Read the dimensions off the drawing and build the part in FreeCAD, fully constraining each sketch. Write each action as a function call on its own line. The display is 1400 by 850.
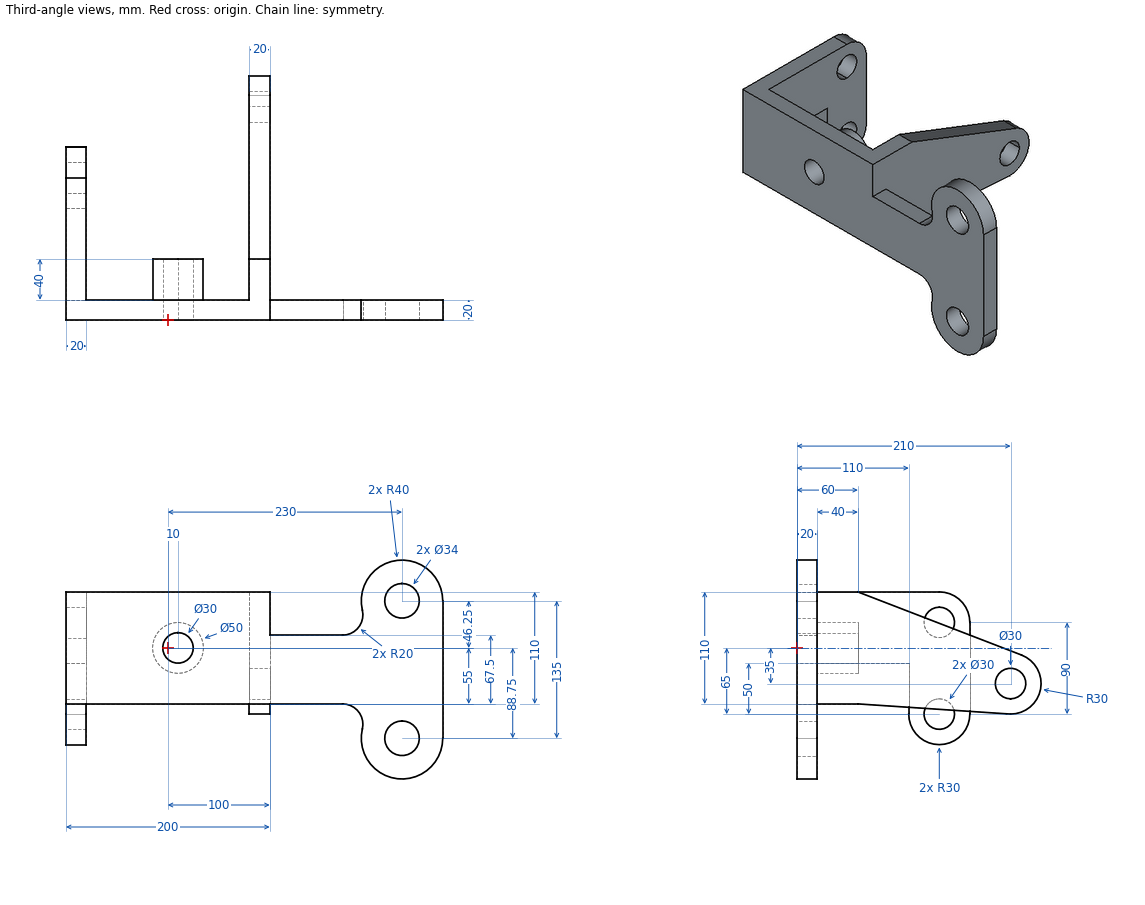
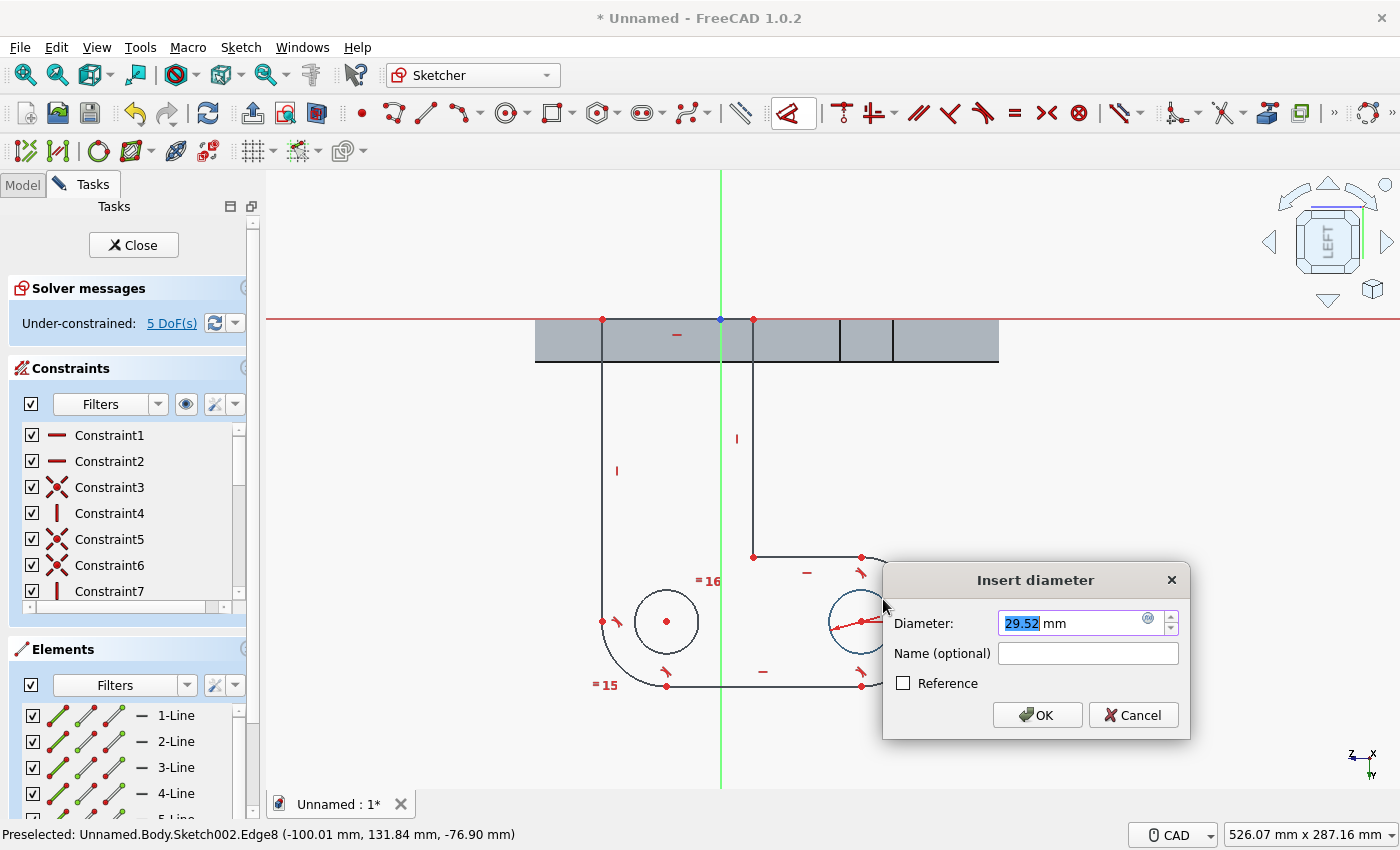
text(30)
key(Return)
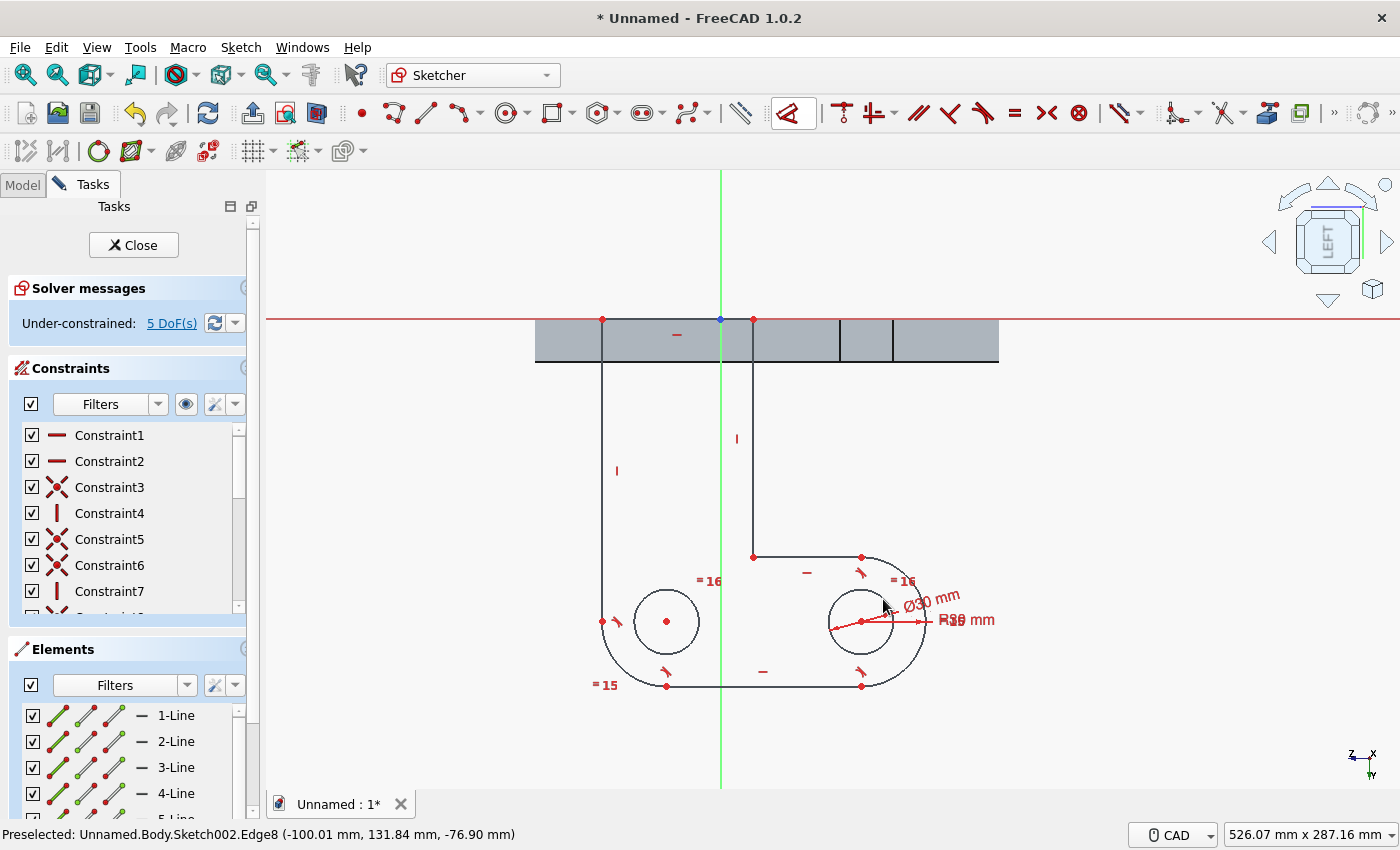
click(753, 319)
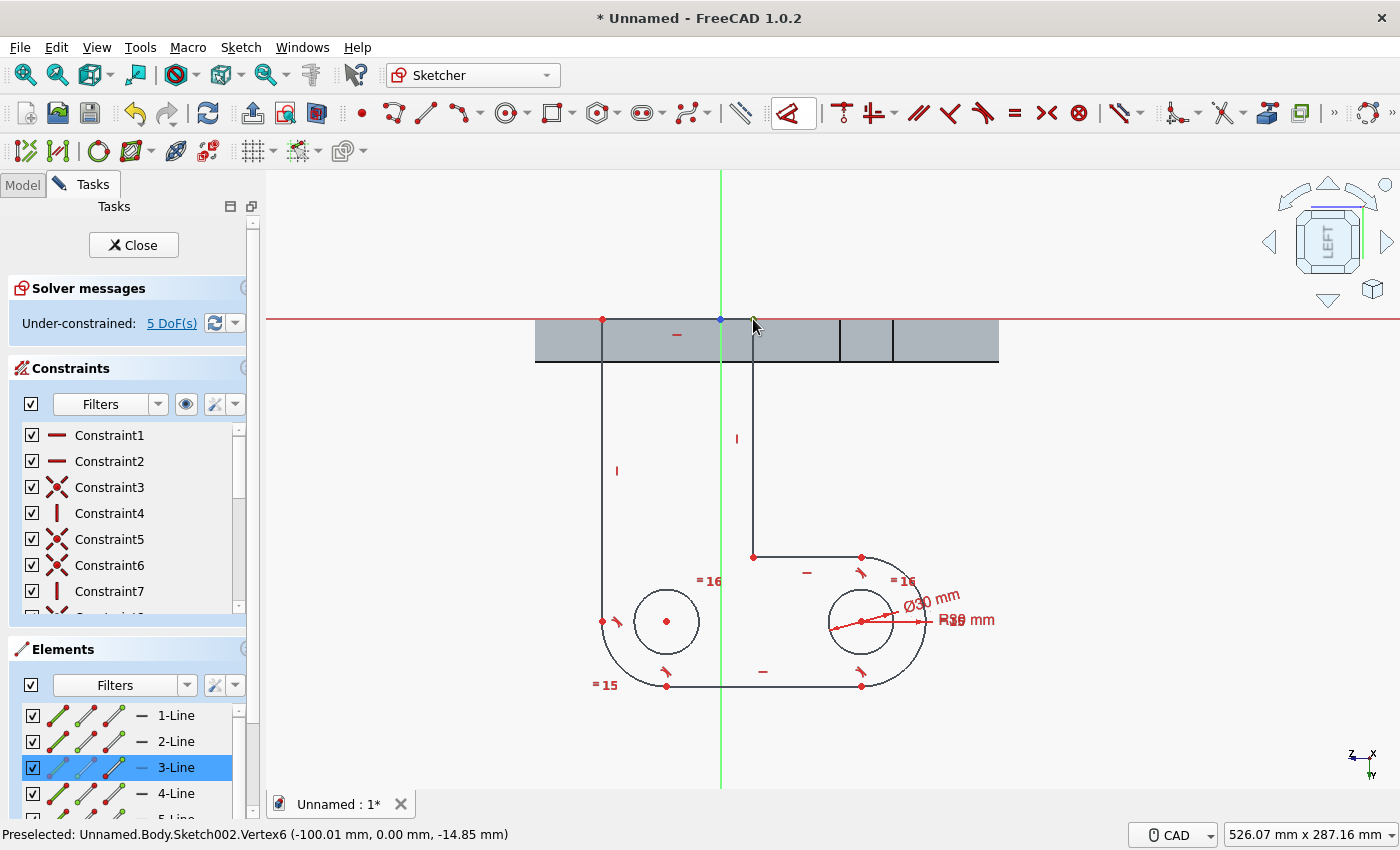
click(361, 319)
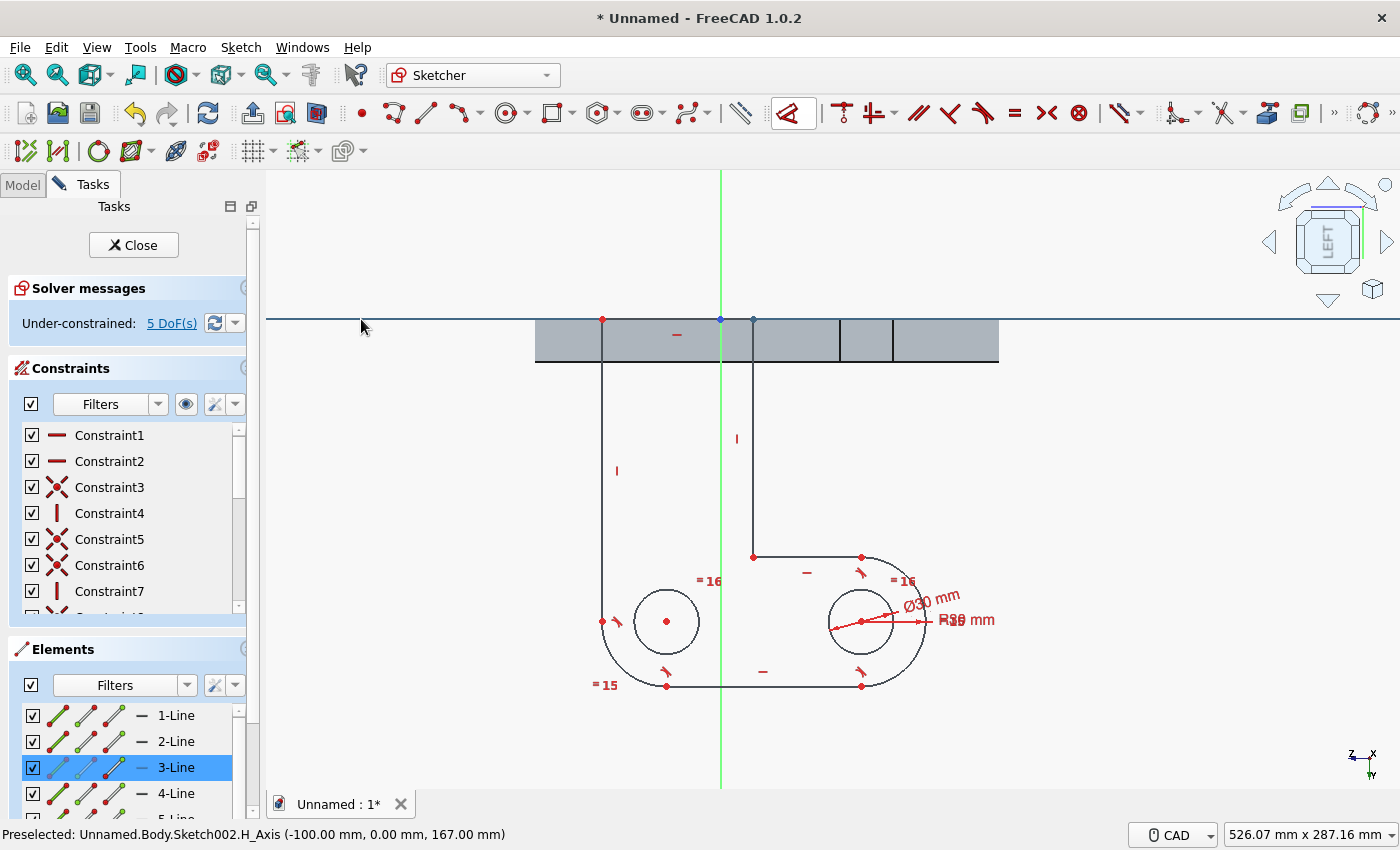
click(842, 114)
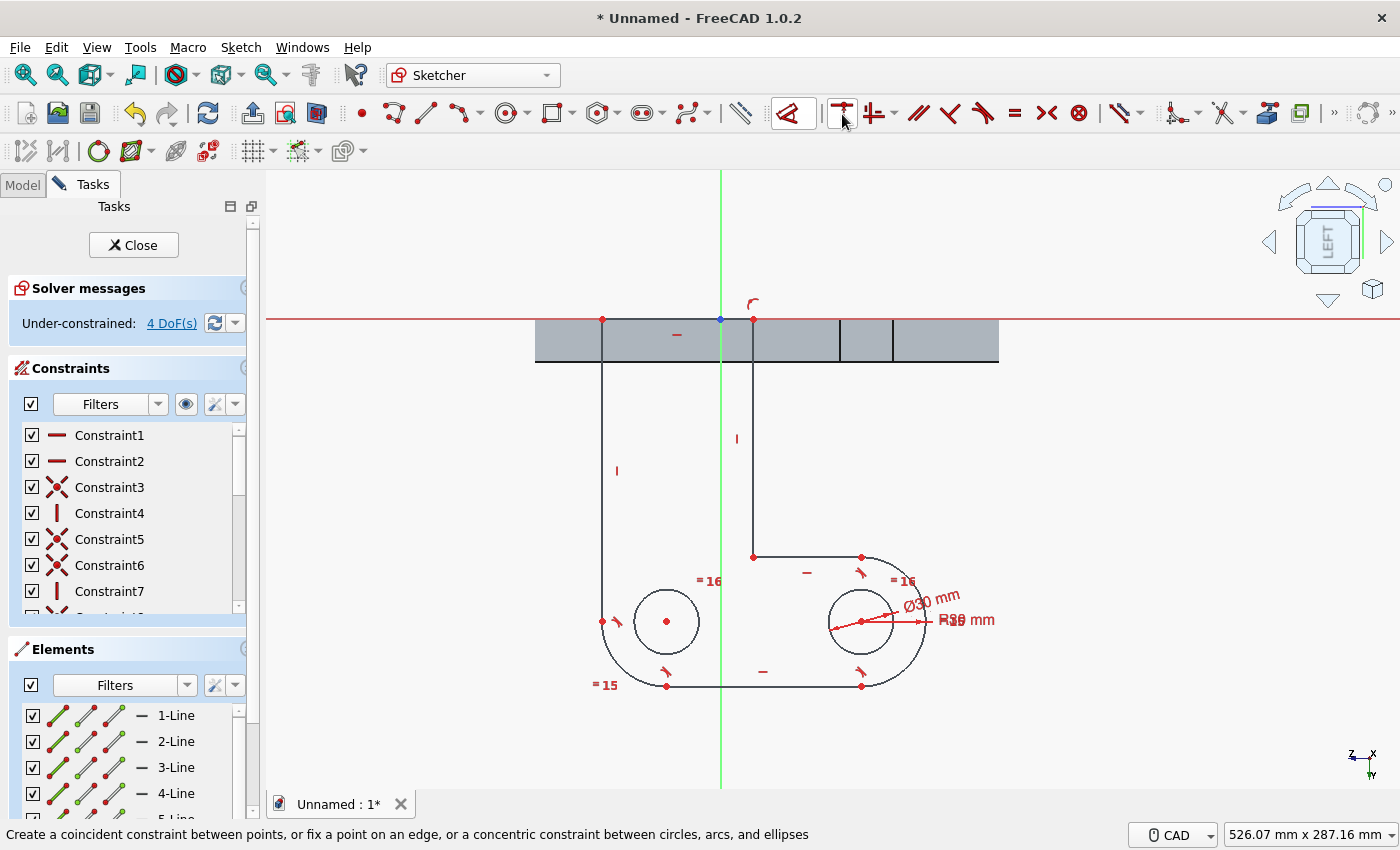
click(725, 687)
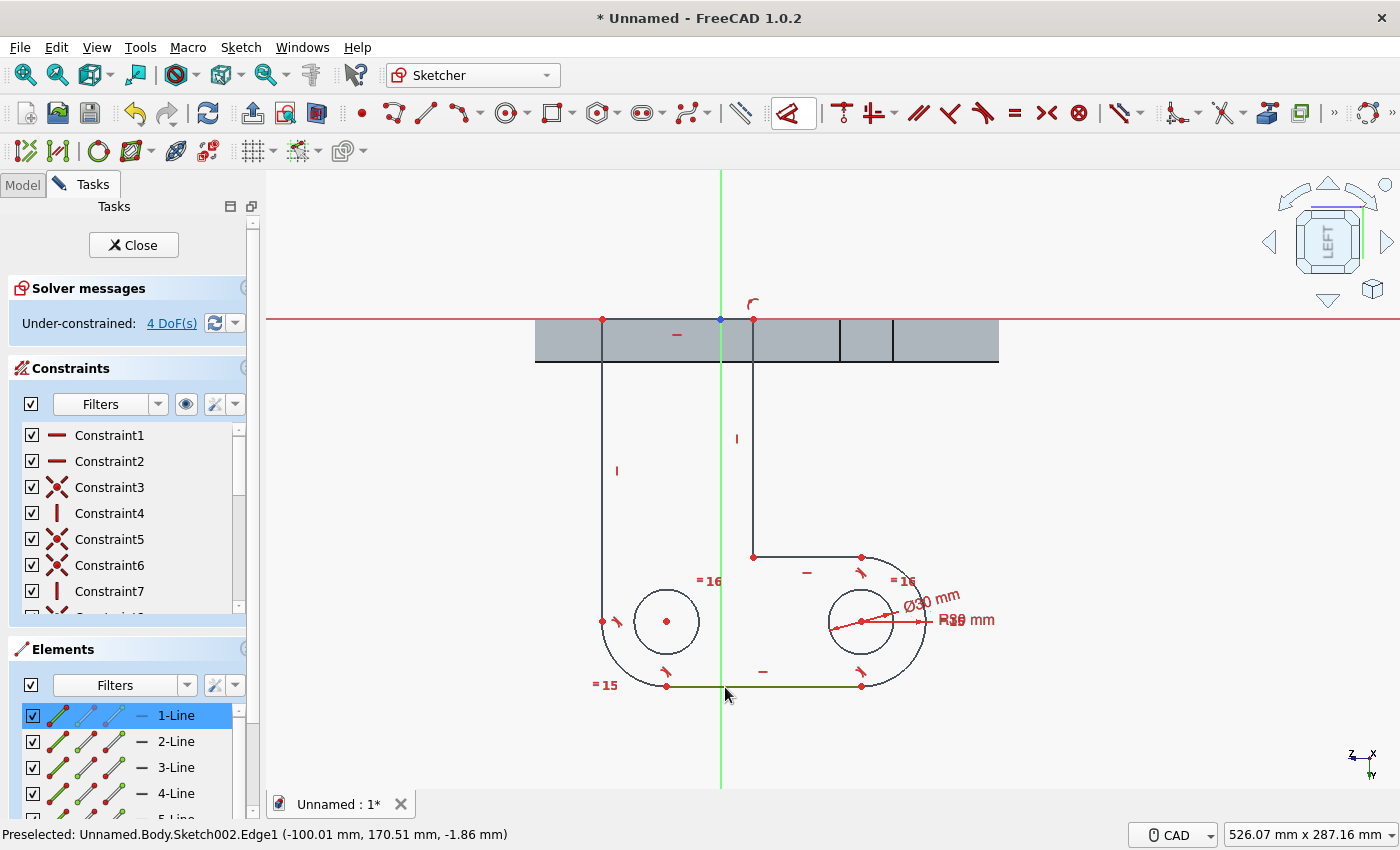
key(l)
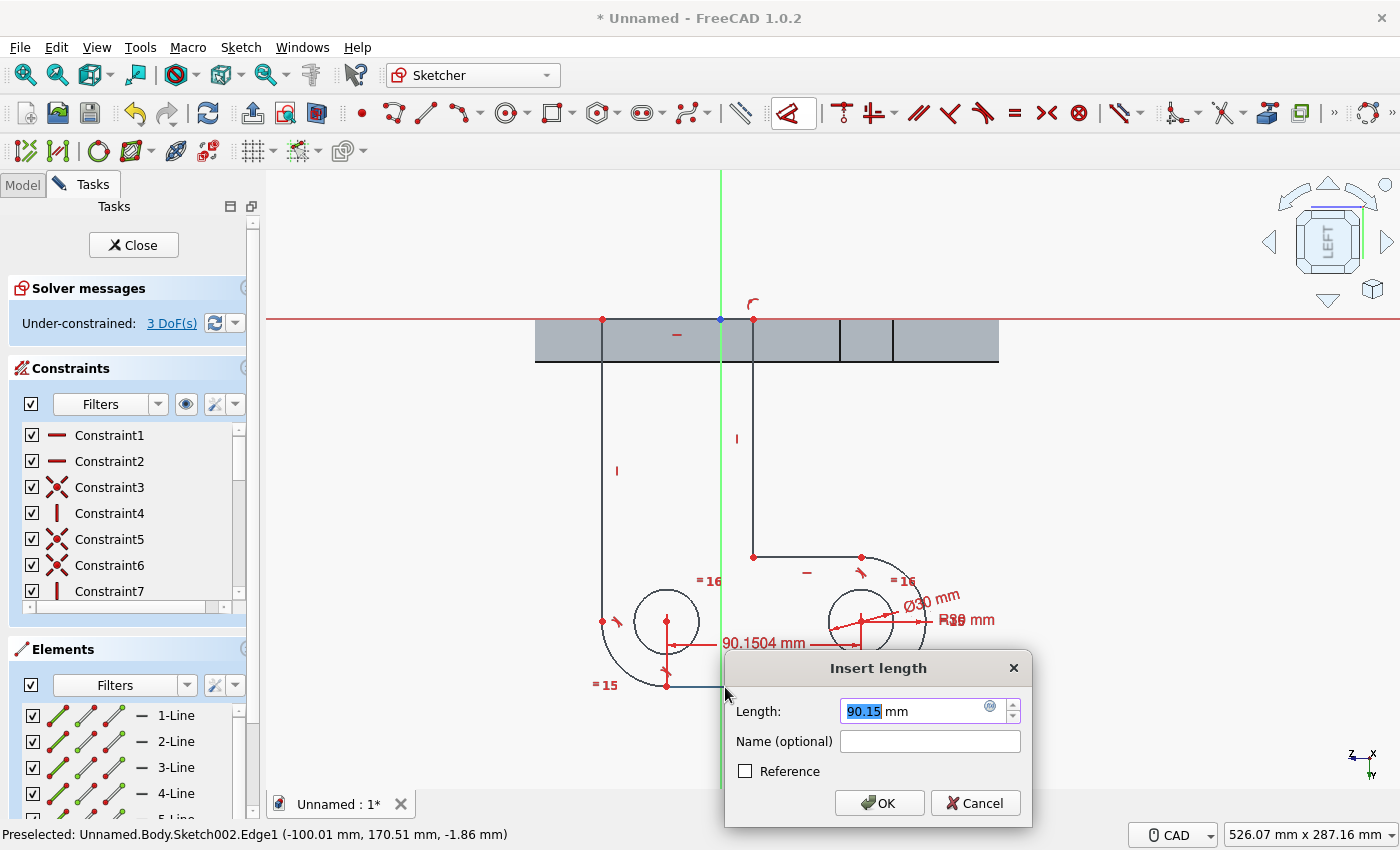
text(90)
key(Return)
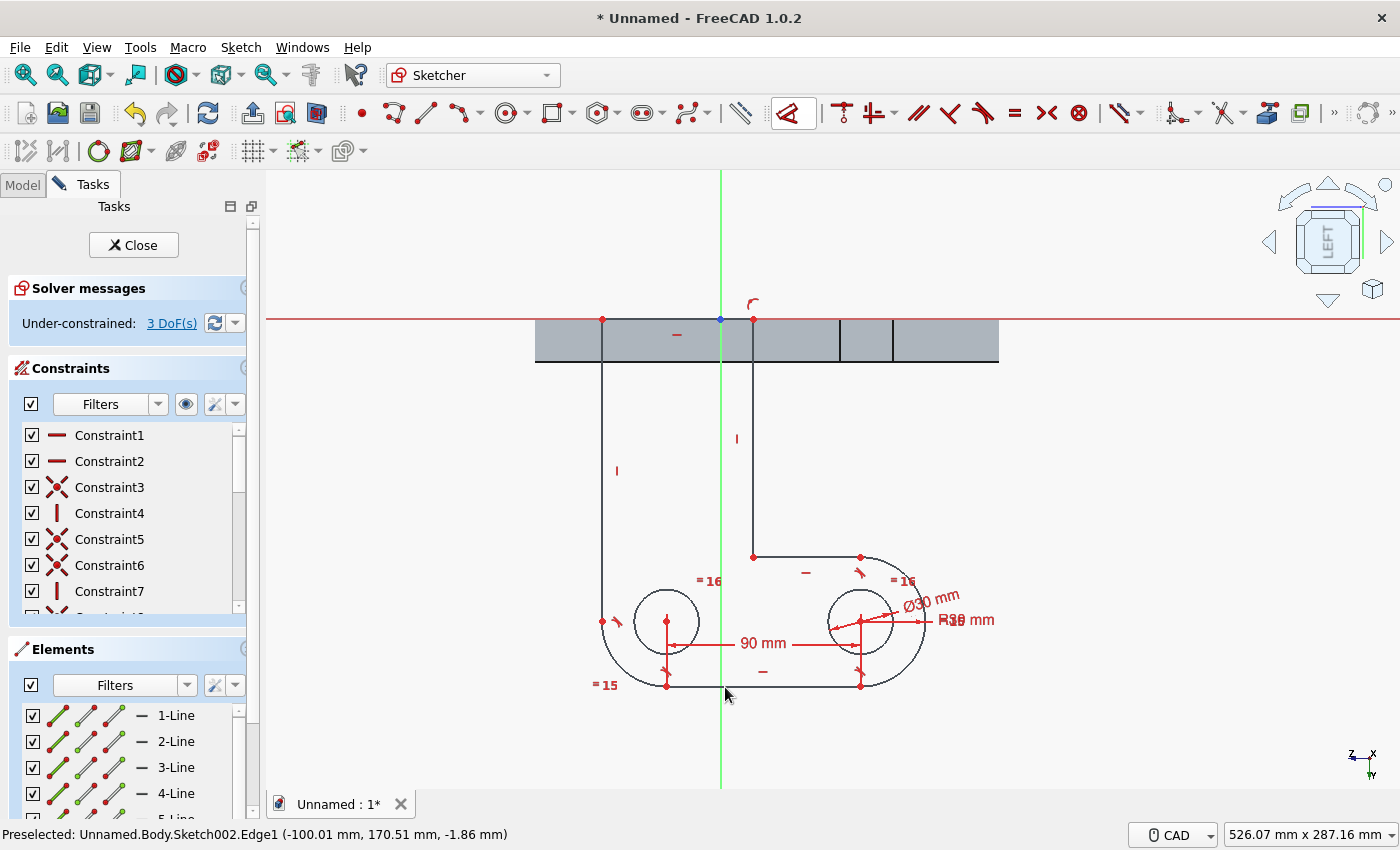
click(828, 557)